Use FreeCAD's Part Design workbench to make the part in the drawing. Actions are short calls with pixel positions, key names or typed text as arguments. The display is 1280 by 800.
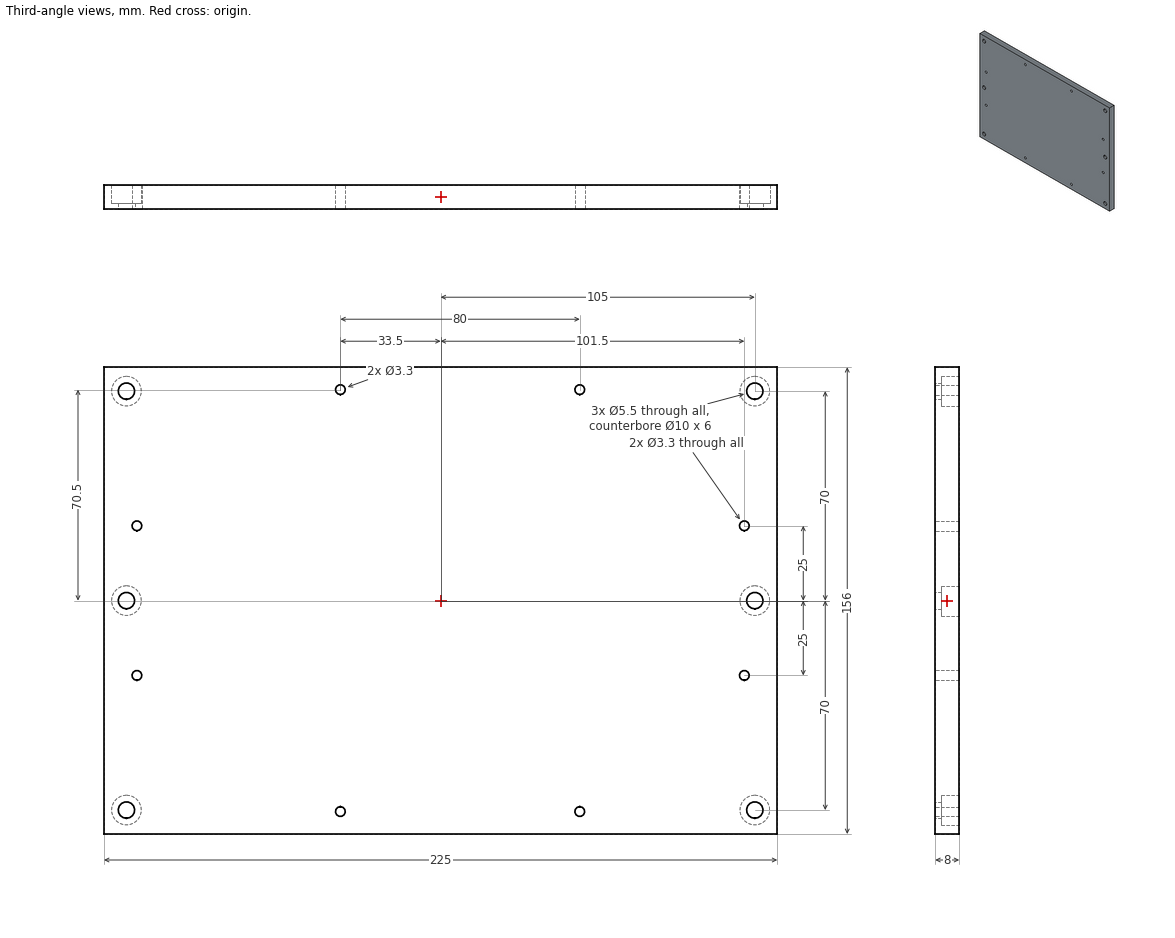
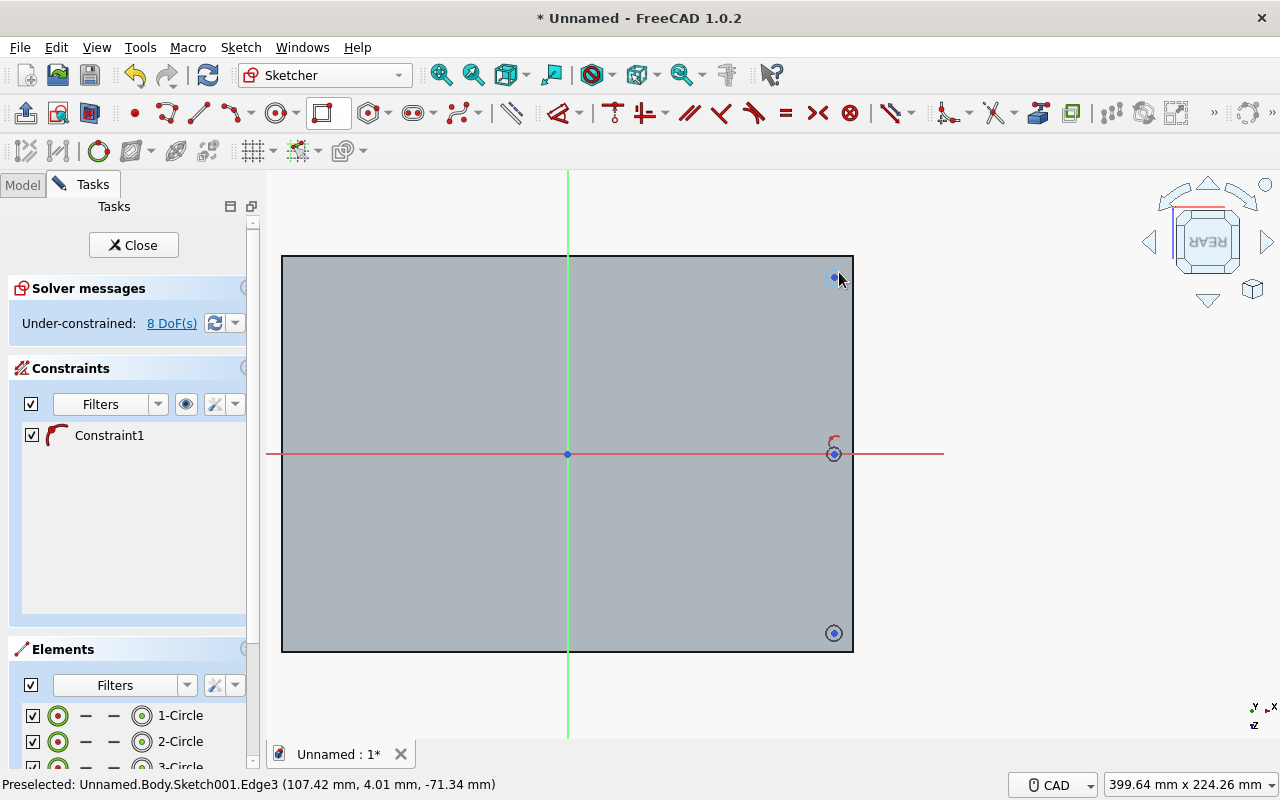
scroll(840, 628, up, 3)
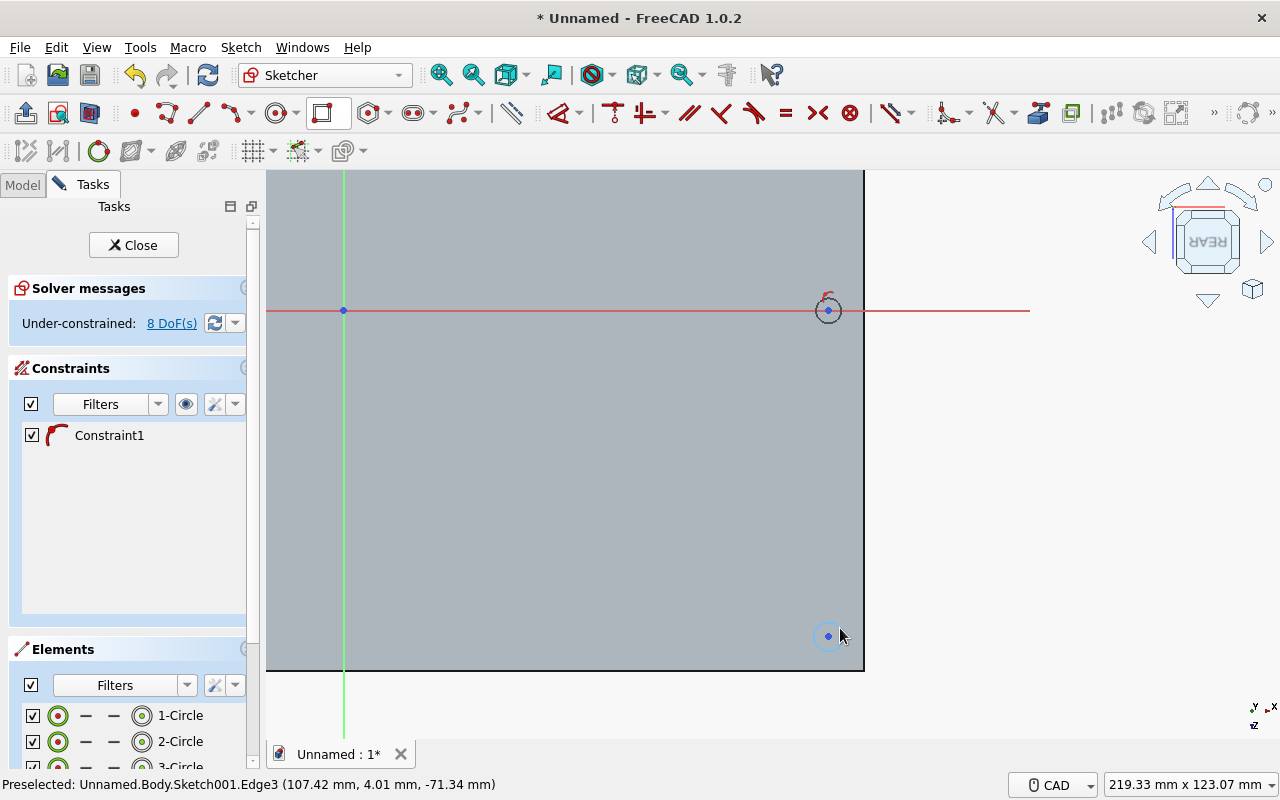
click(839, 627)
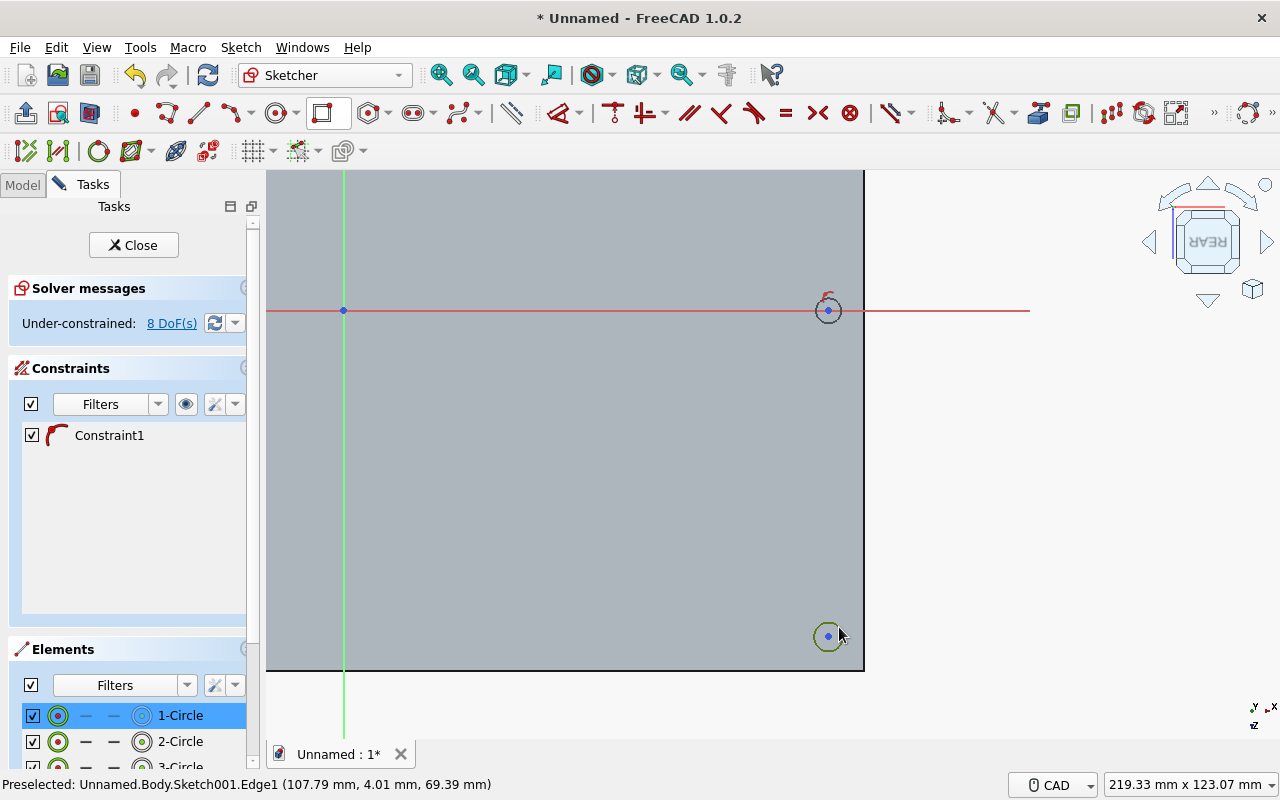
click(816, 311)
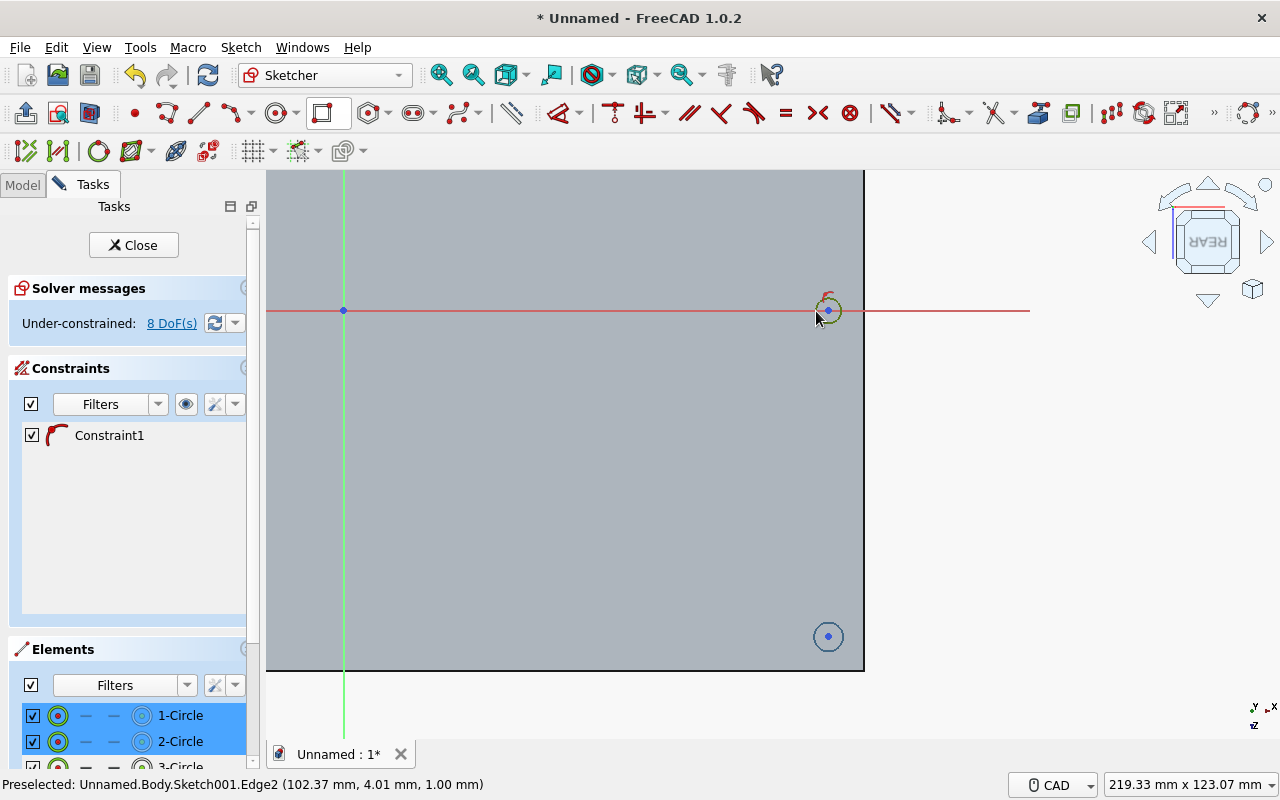
scroll(840, 629, down, 3)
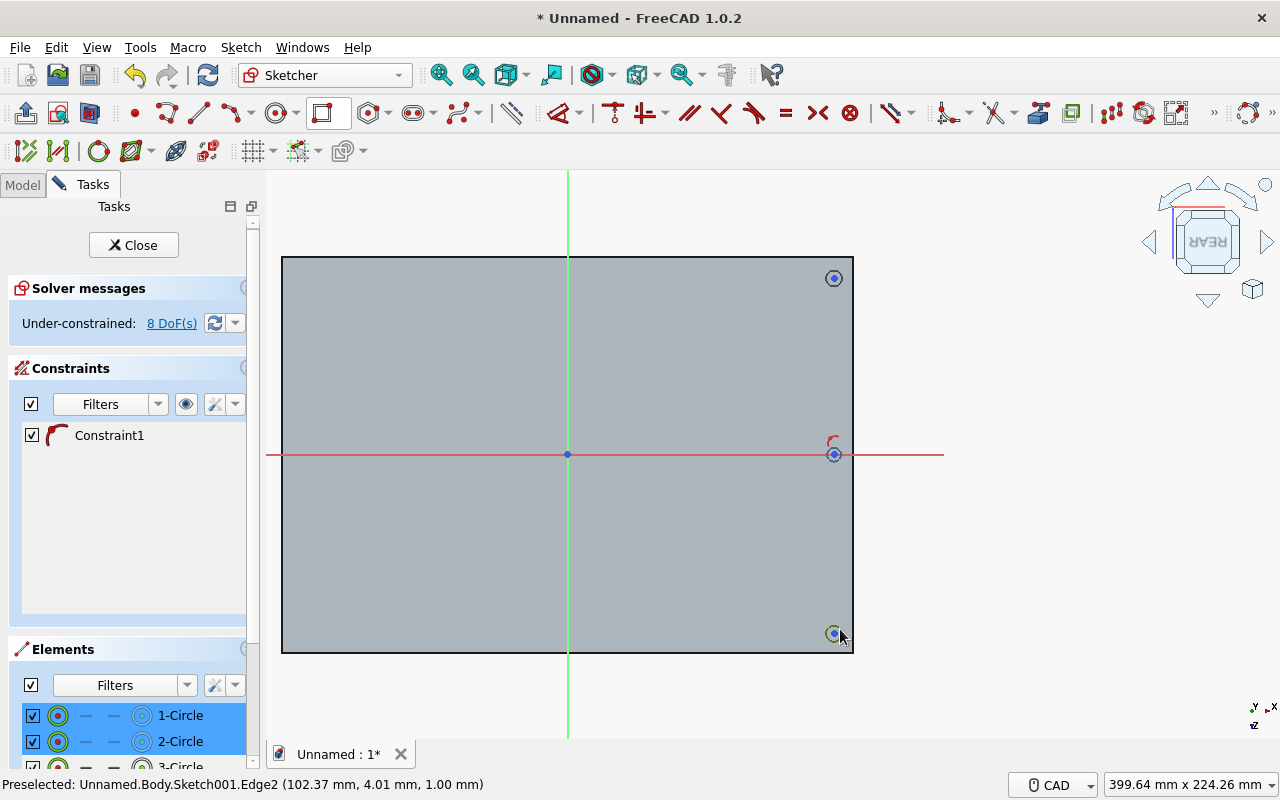
scroll(840, 273, up, 3)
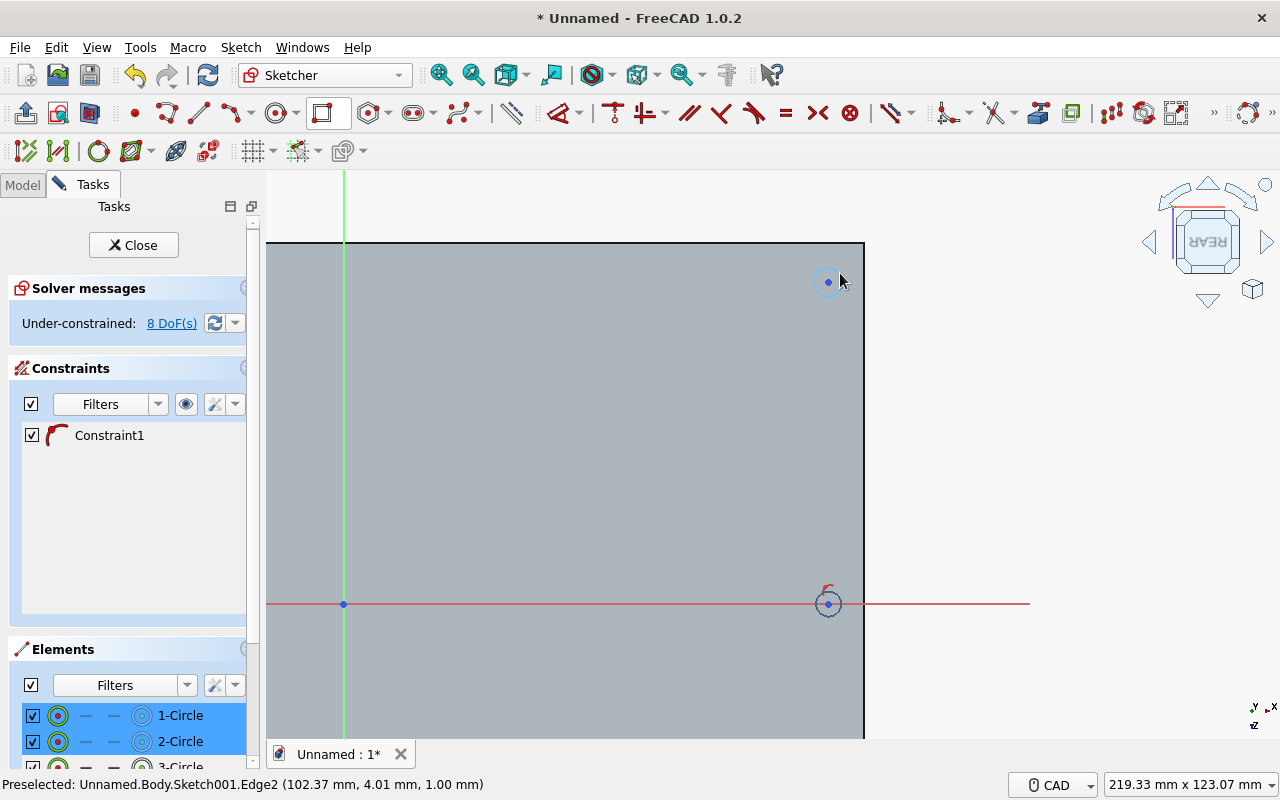
click(839, 272)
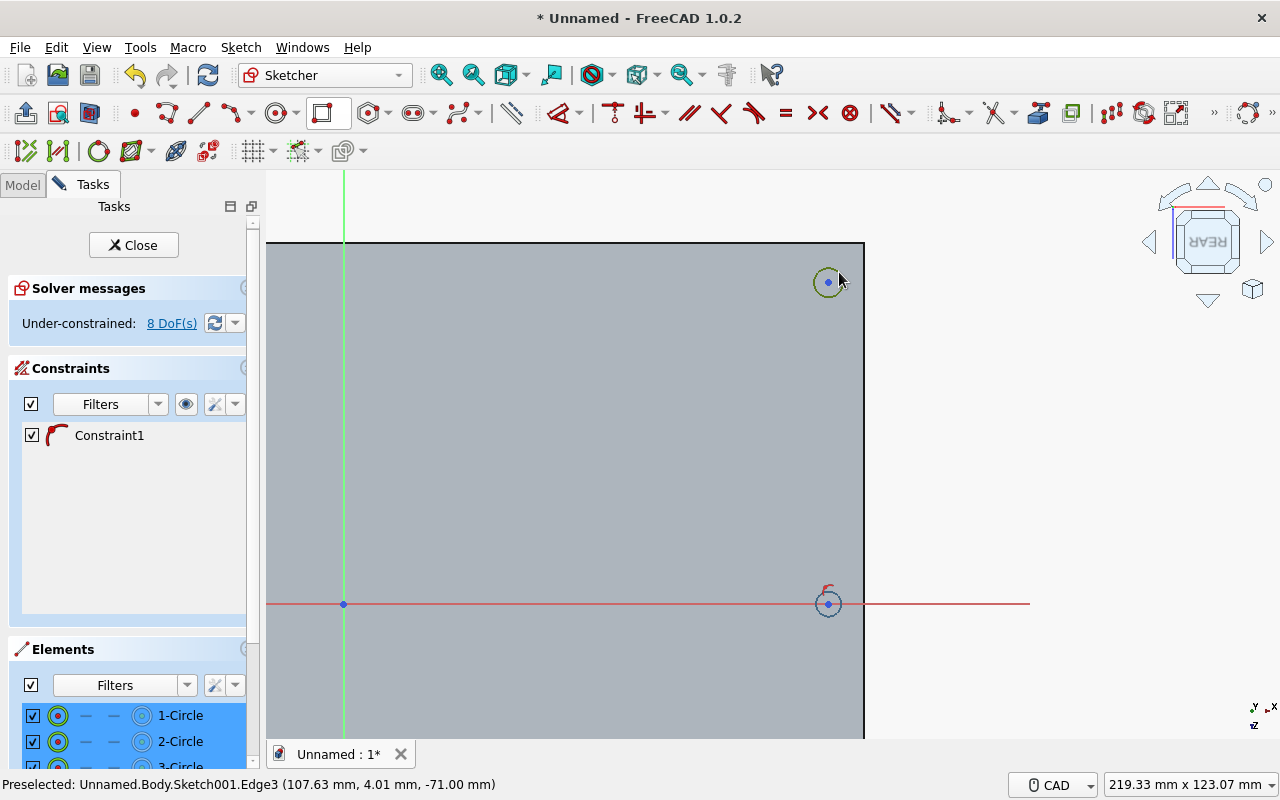
click(786, 114)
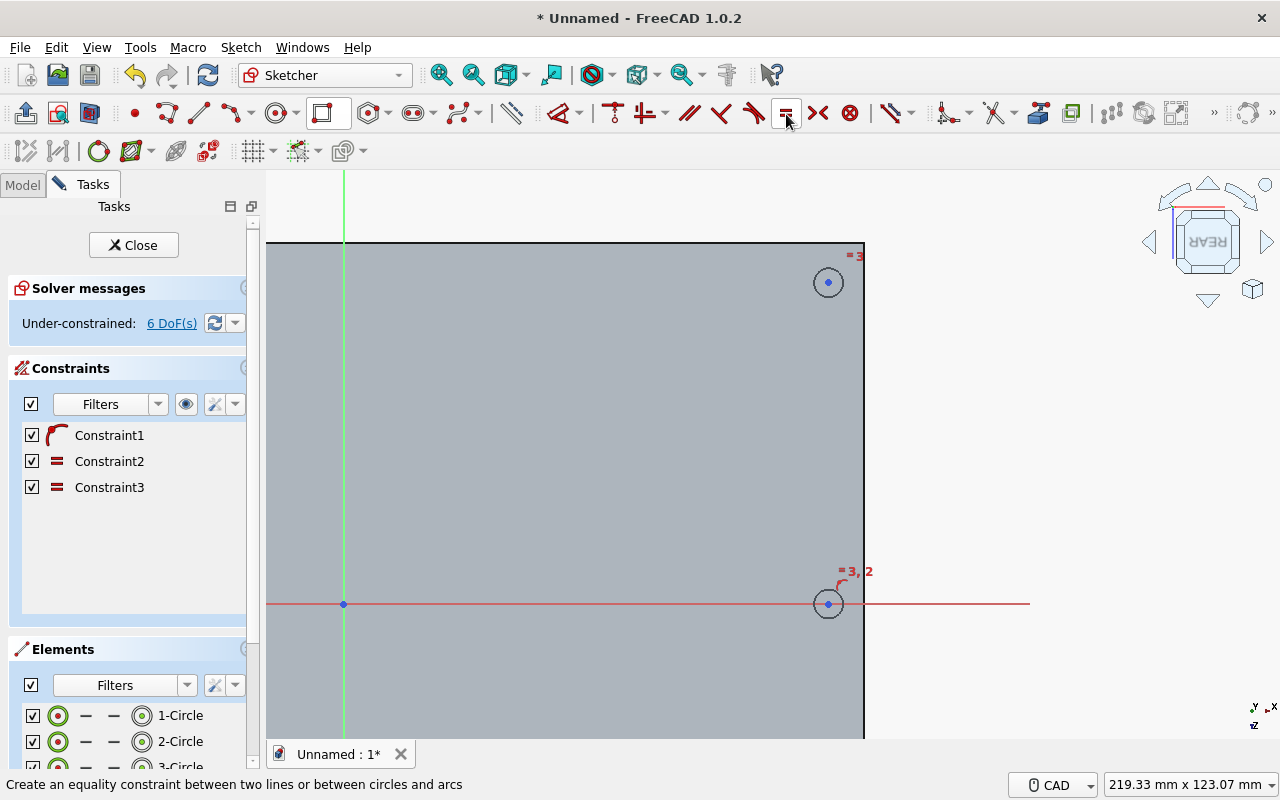
scroll(840, 273, down, 3)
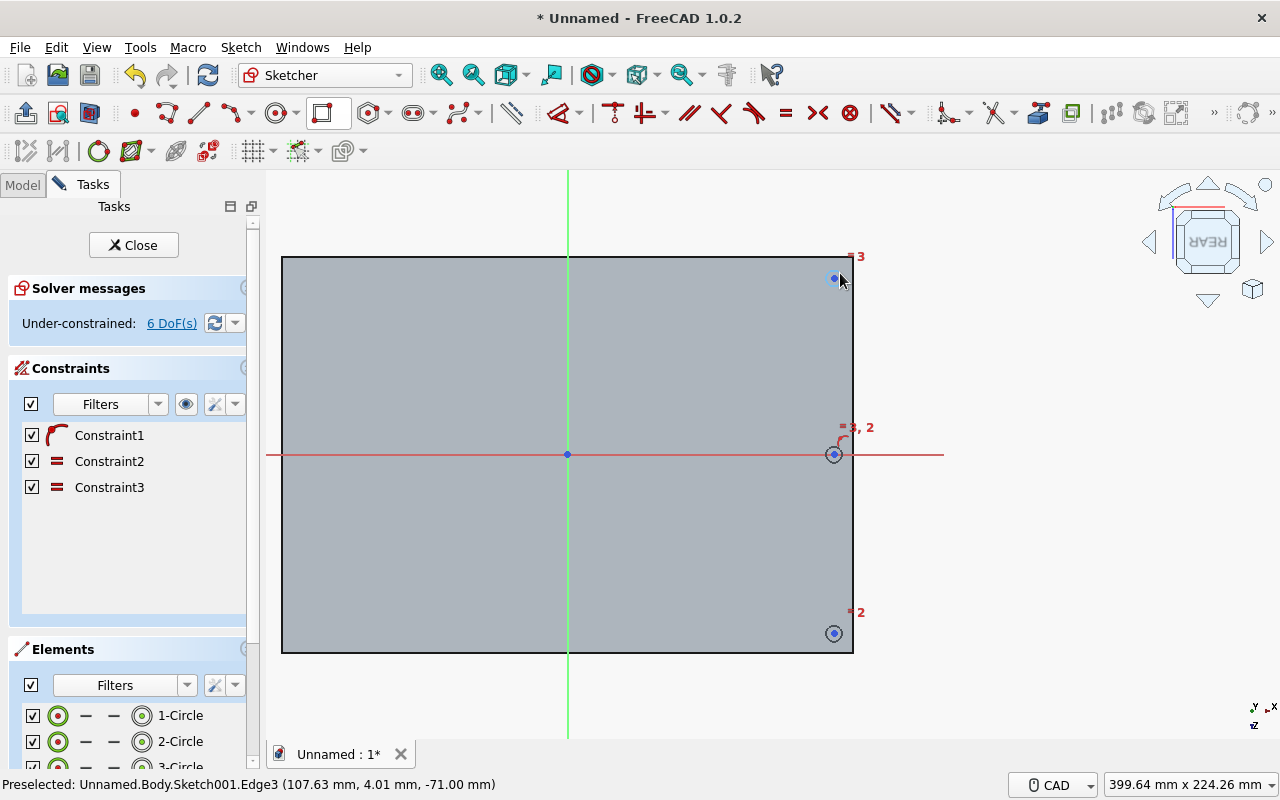
click(834, 634)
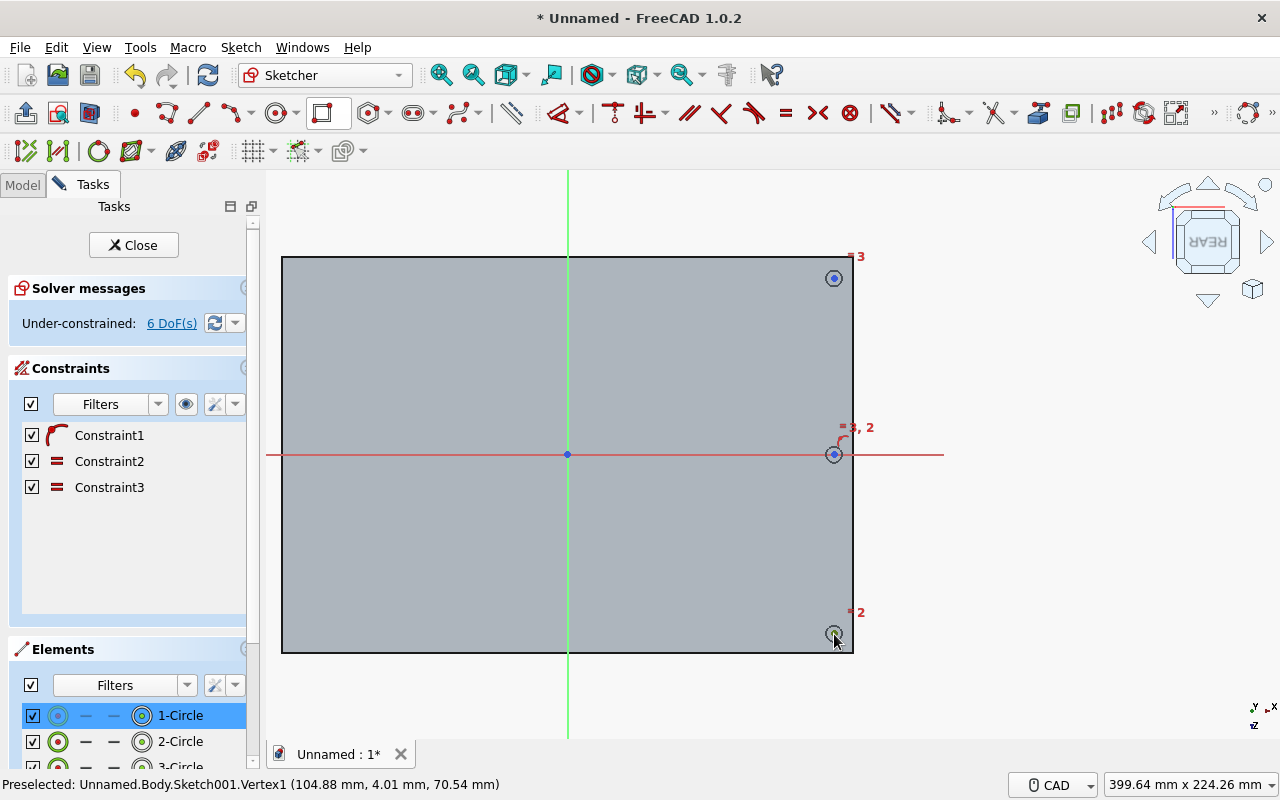
click(834, 455)